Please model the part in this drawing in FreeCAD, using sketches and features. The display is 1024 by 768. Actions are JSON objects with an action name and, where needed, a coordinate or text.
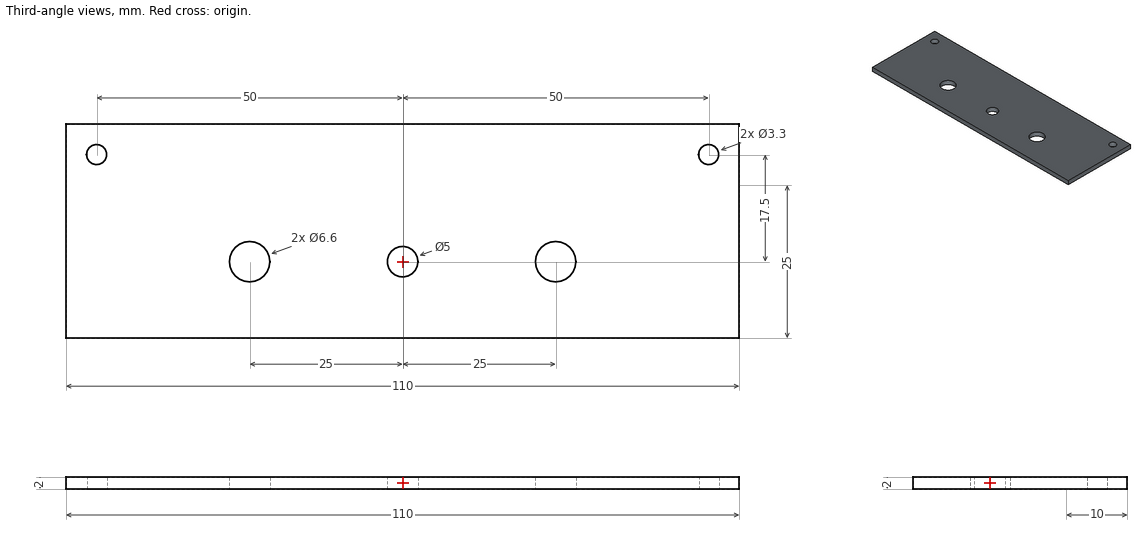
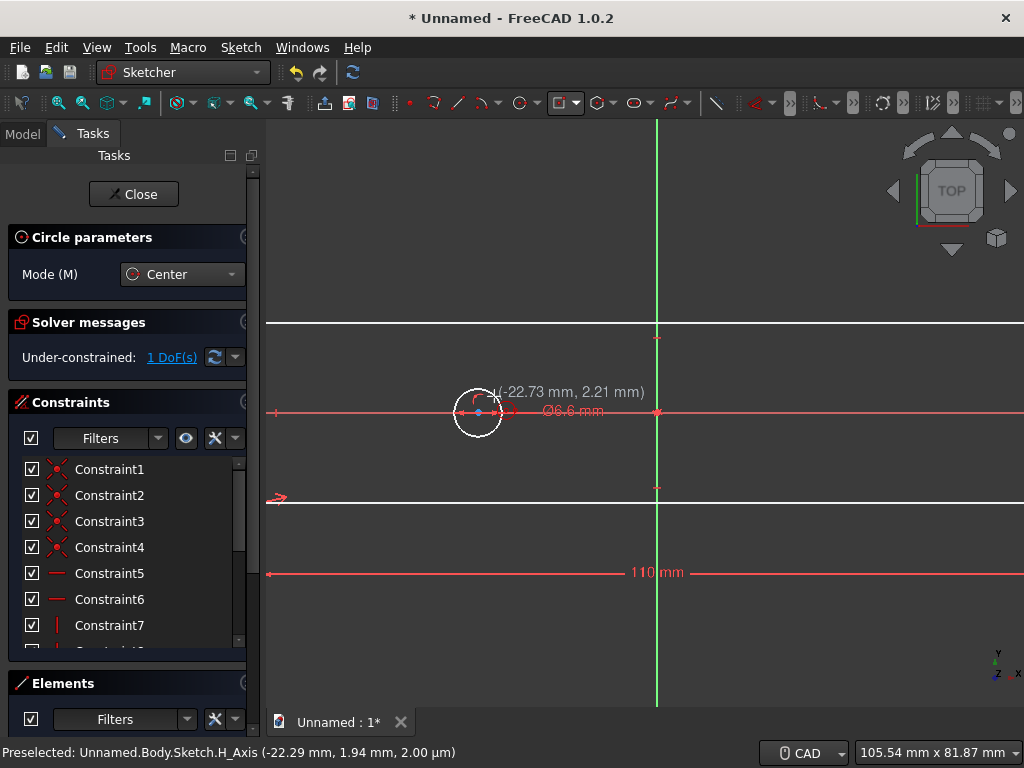
{"action": "left_click", "coordinate": [837, 413]}
{"action": "mouse_move", "coordinate": [854, 396]}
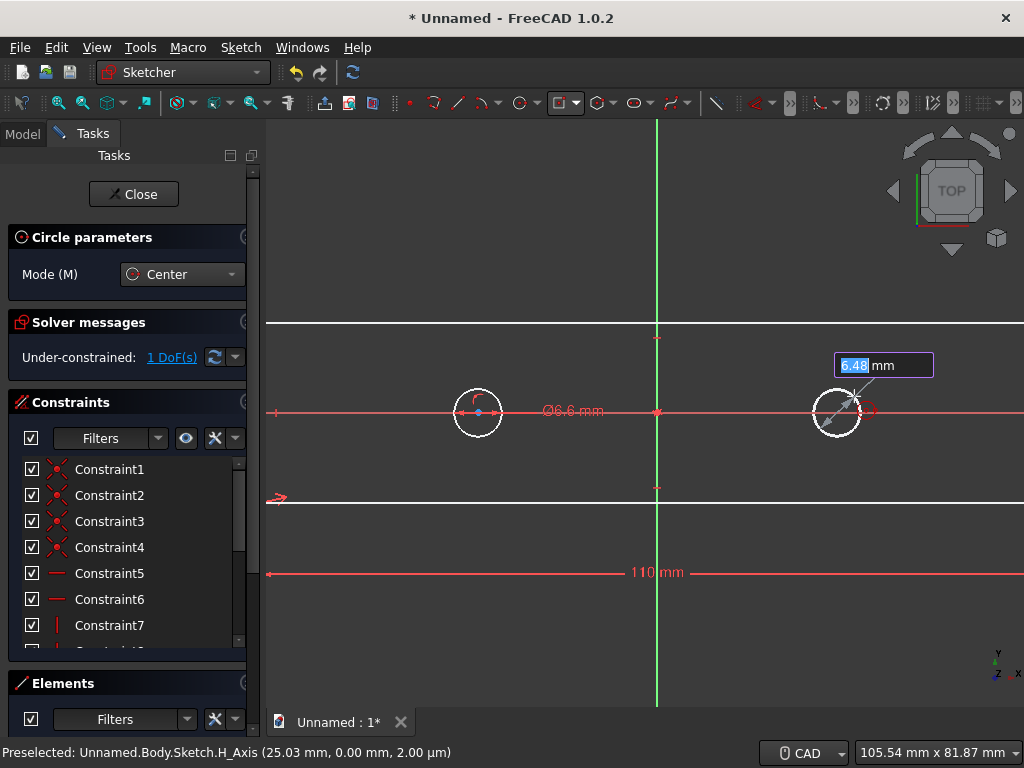
{"action": "type", "text": "6.6"}
{"action": "key", "text": "Return"}
{"action": "key", "text": "Escape"}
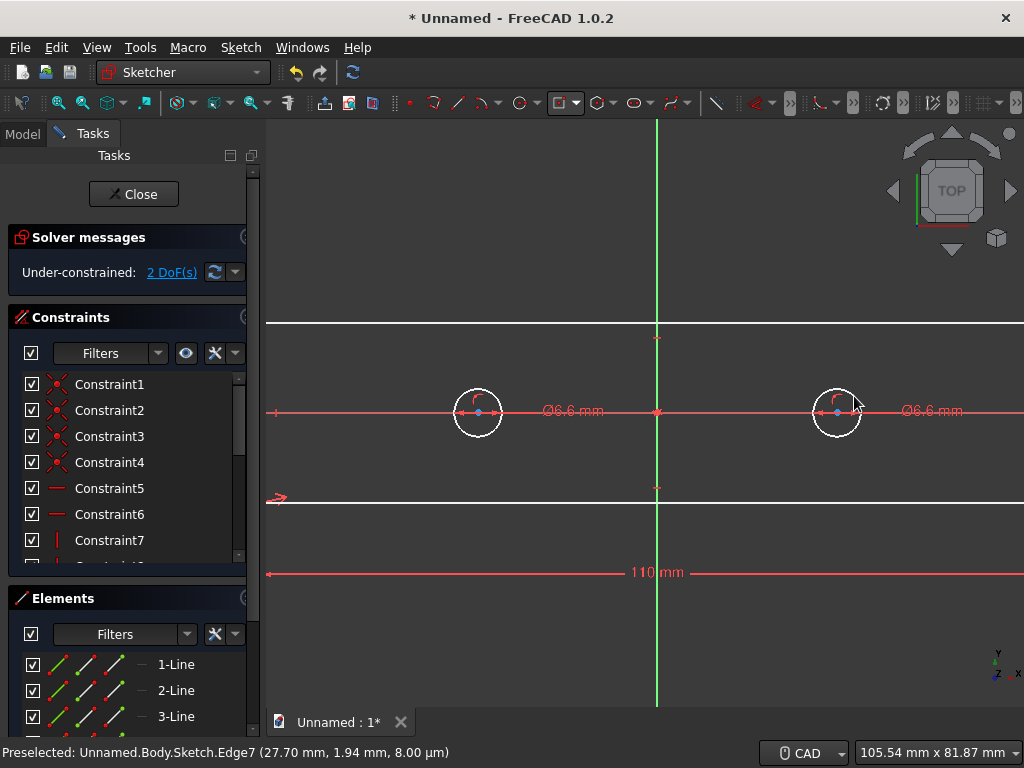
{"action": "left_click", "coordinate": [756, 104]}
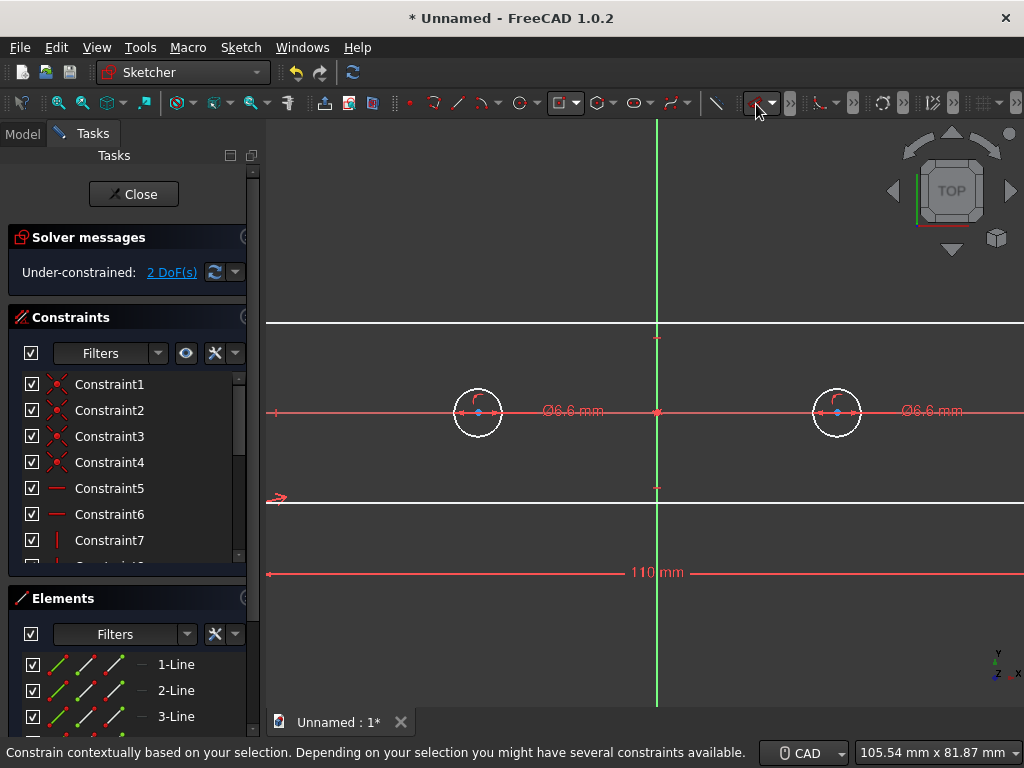
{"action": "left_click", "coordinate": [478, 413]}
{"action": "left_click", "coordinate": [568, 447]}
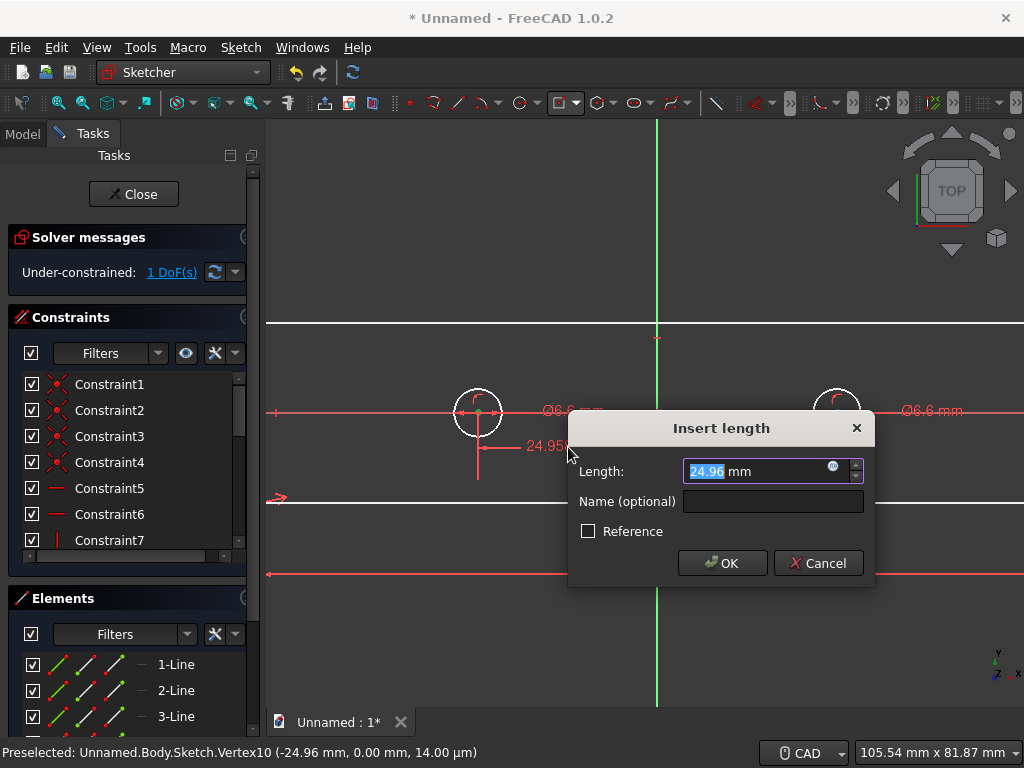
{"action": "type", "text": "25"}
{"action": "key", "text": "Return"}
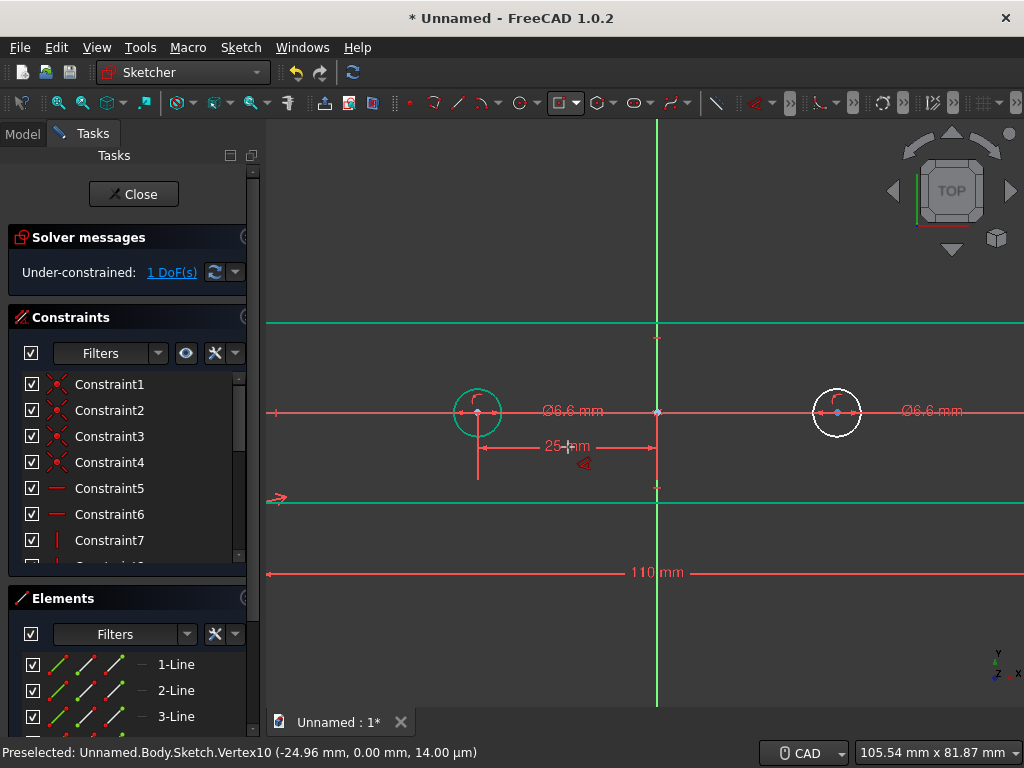
{"action": "left_click", "coordinate": [837, 413]}
{"action": "left_click", "coordinate": [747, 447]}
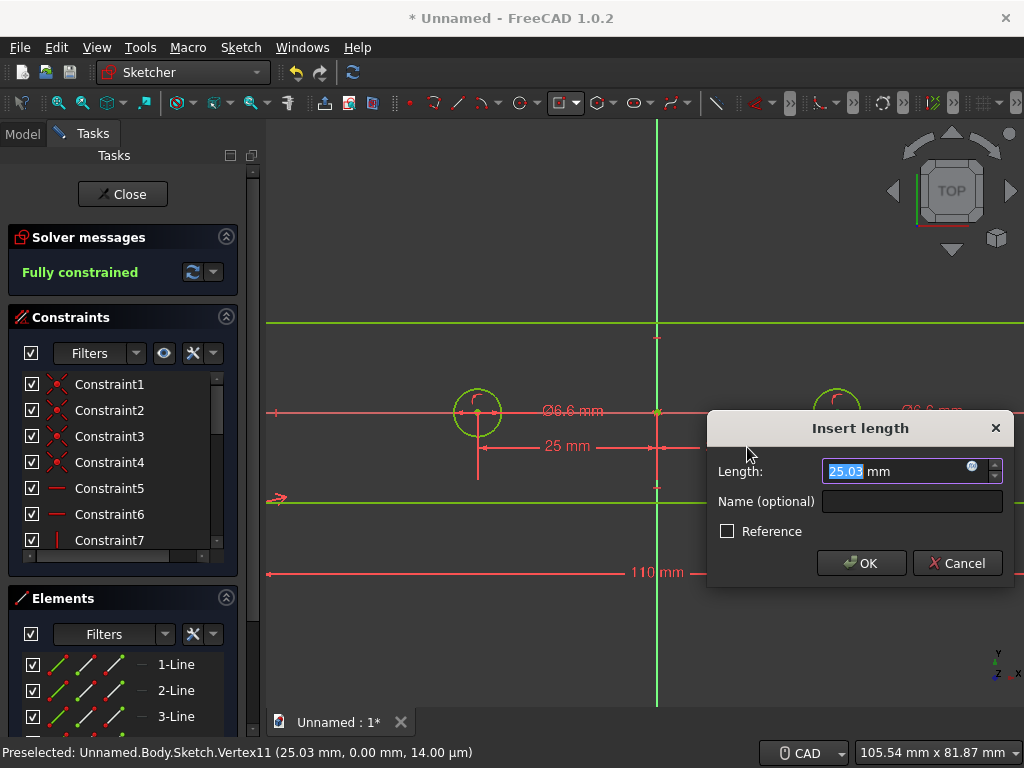
{"action": "type", "text": "25"}
{"action": "key", "text": "Return"}
{"action": "key", "text": "Escape"}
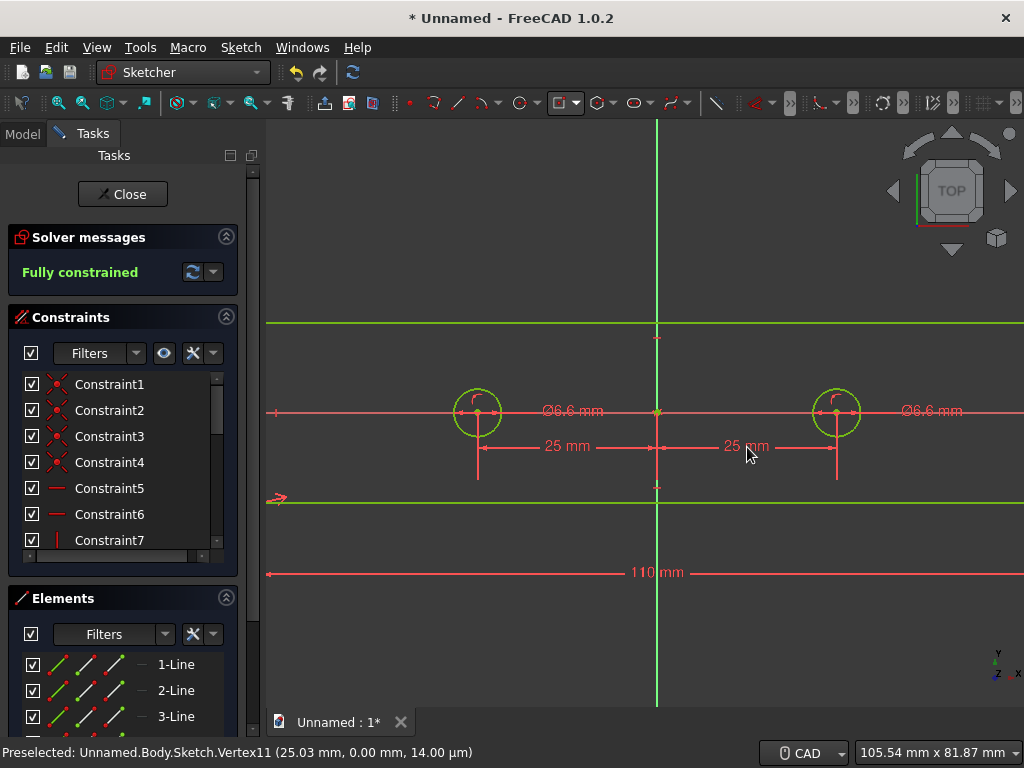
{"action": "left_click", "coordinate": [123, 194]}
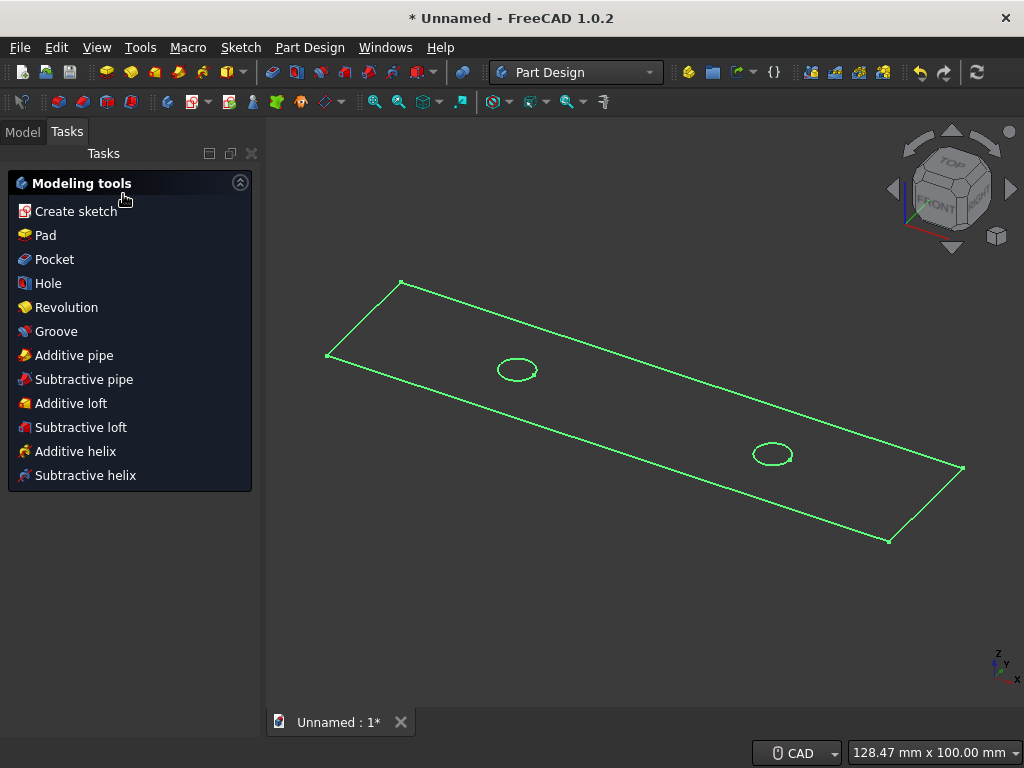
{"action": "left_click", "coordinate": [108, 72]}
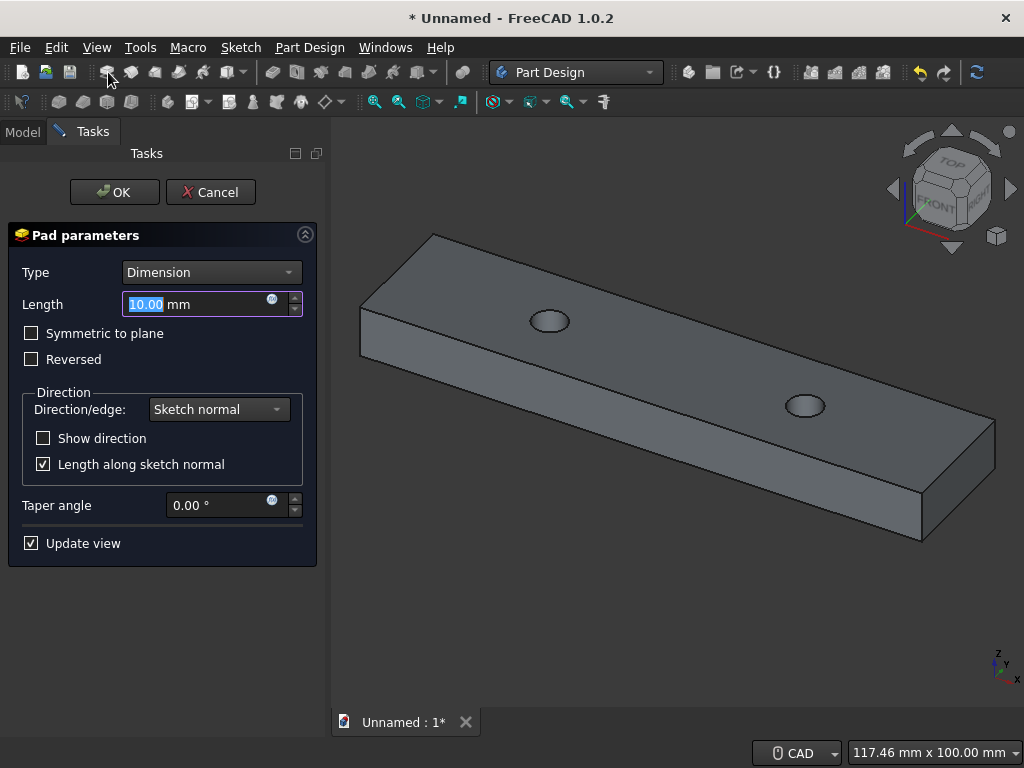
{"action": "type", "text": "2"}
{"action": "key", "text": "Tab"}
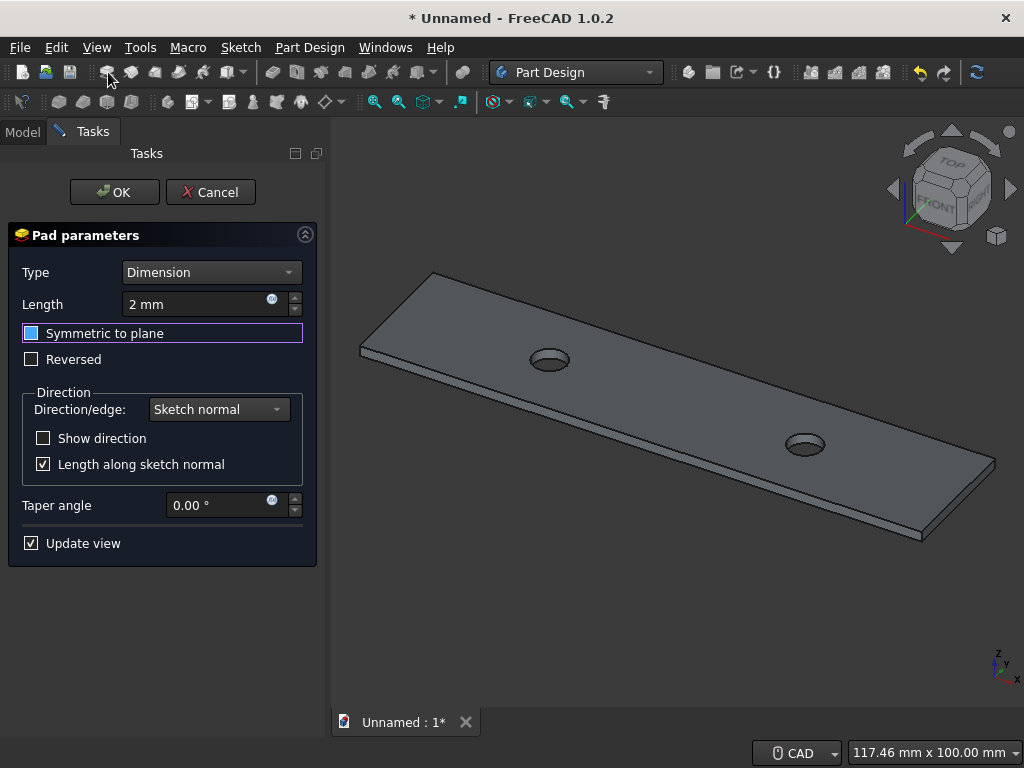
{"action": "left_click", "coordinate": [30, 333]}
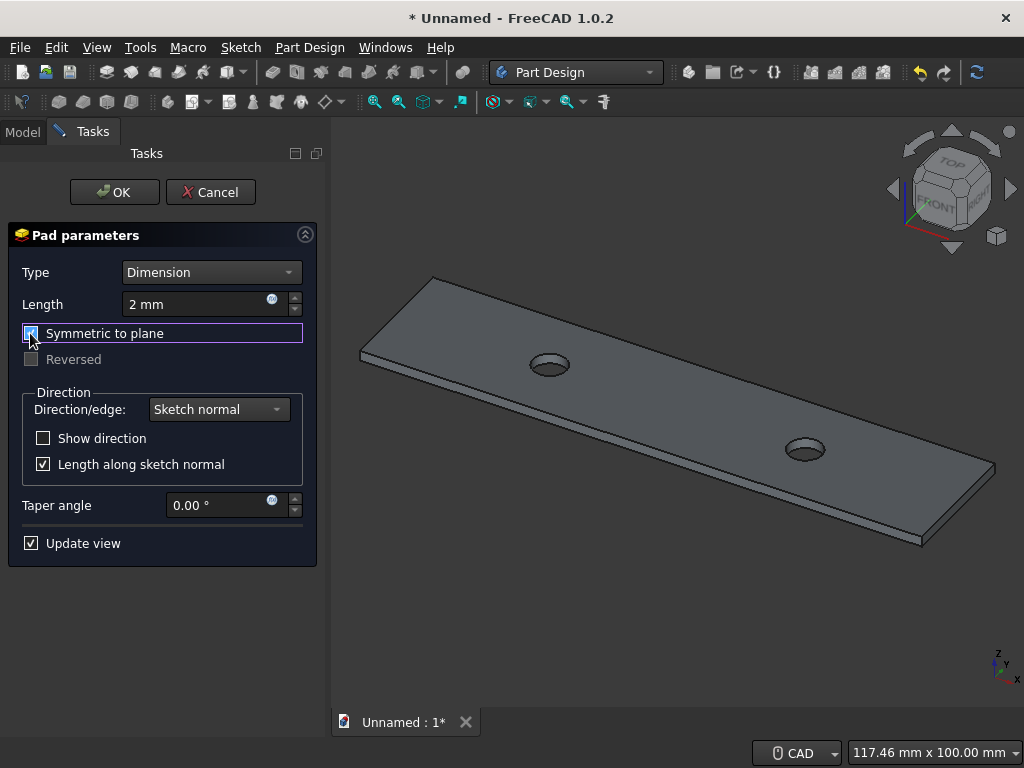
{"action": "left_click", "coordinate": [115, 192]}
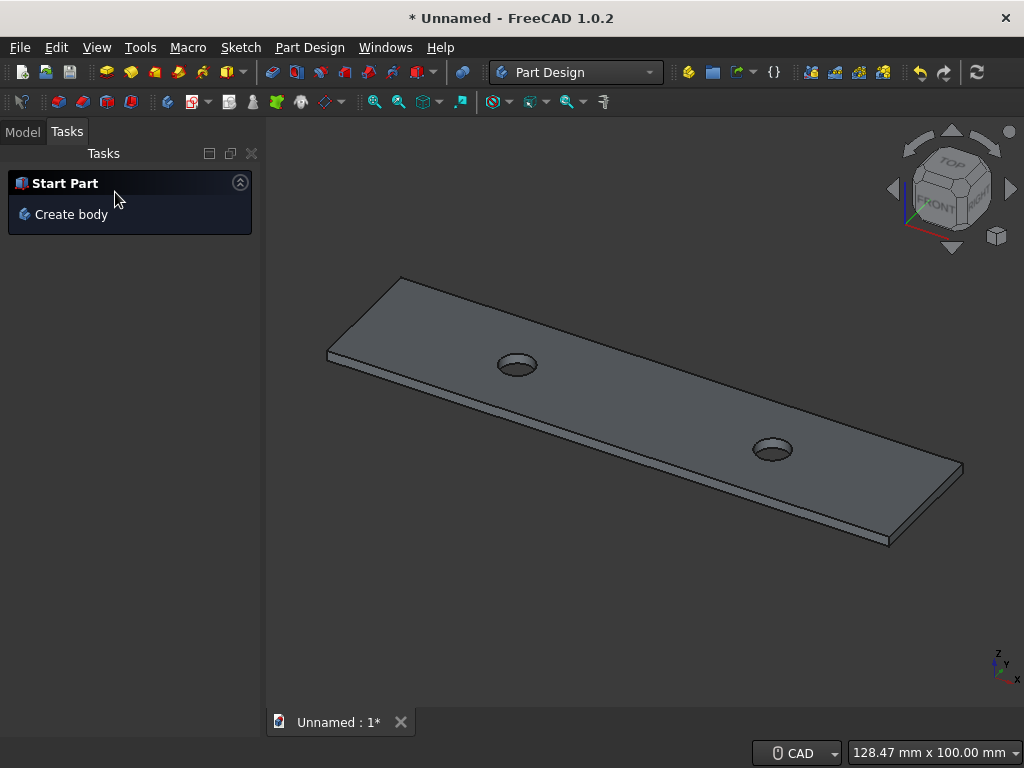
{"action": "left_click", "coordinate": [645, 406]}